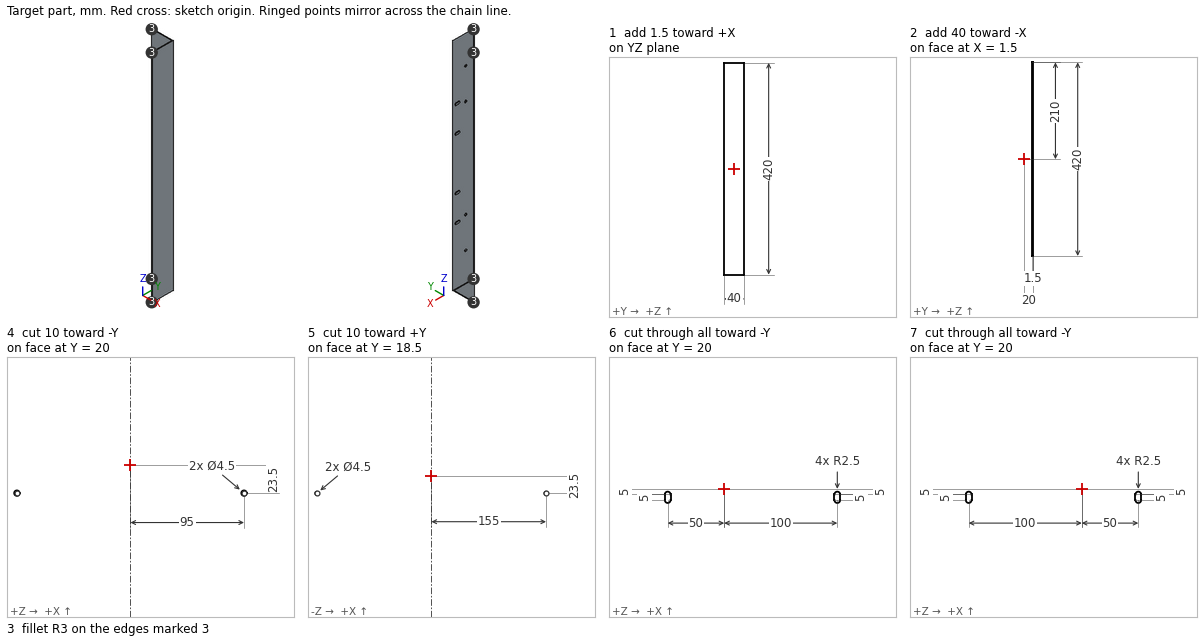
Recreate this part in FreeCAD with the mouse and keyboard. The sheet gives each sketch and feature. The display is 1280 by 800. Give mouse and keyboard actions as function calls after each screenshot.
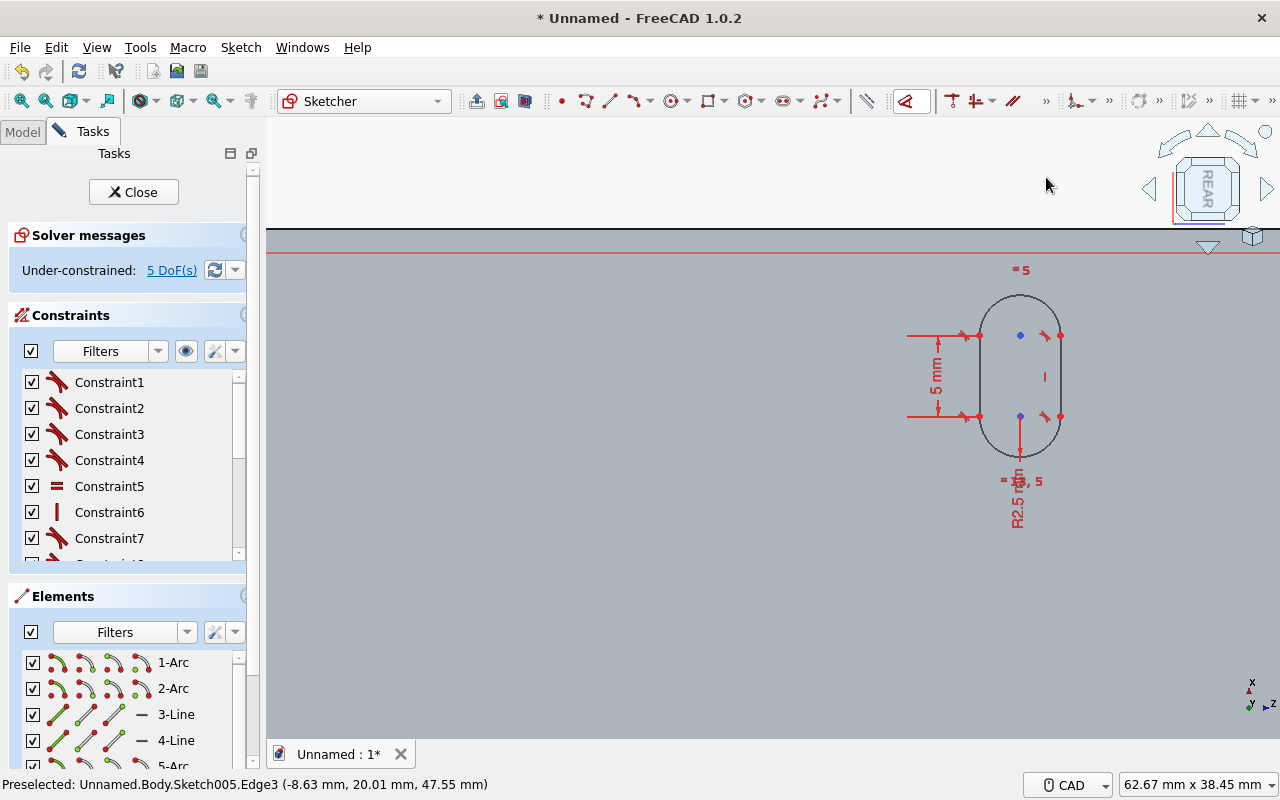
scroll(999, 452, down, 7)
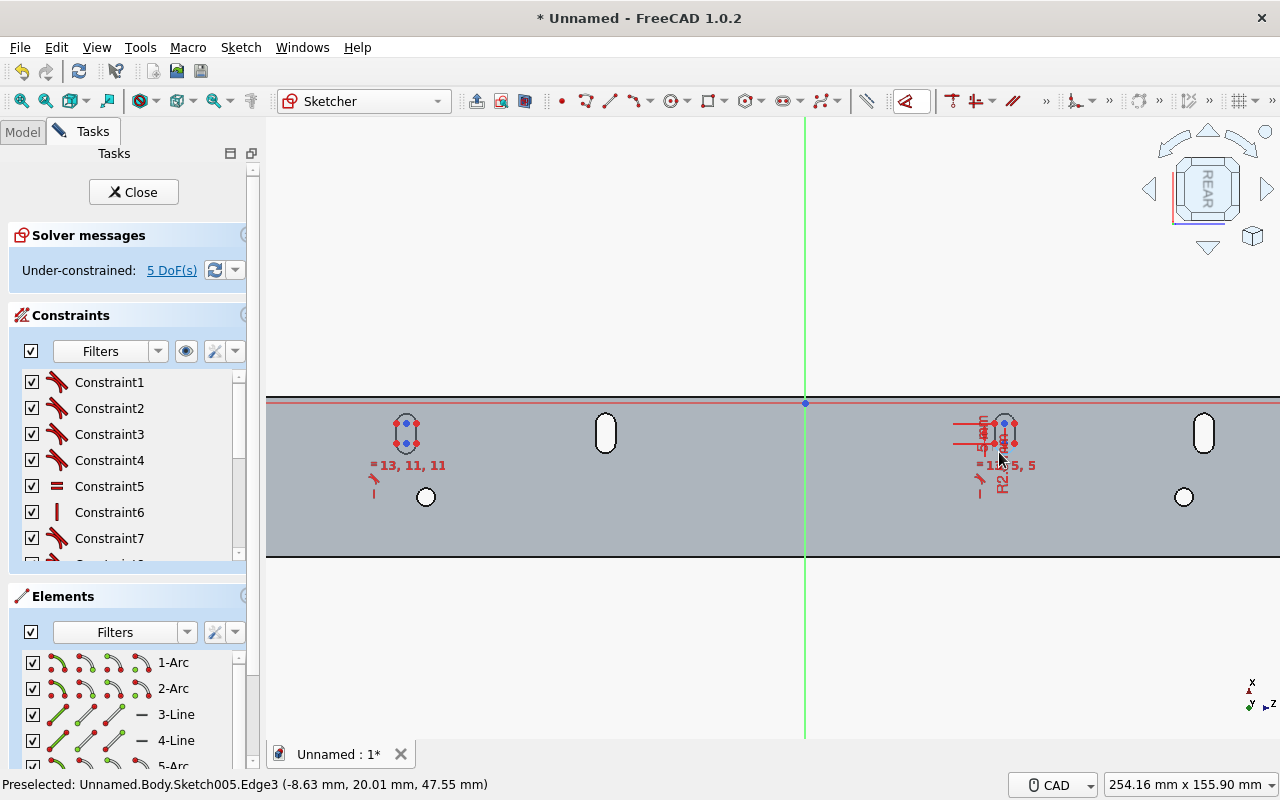
scroll(396, 438, up, 5)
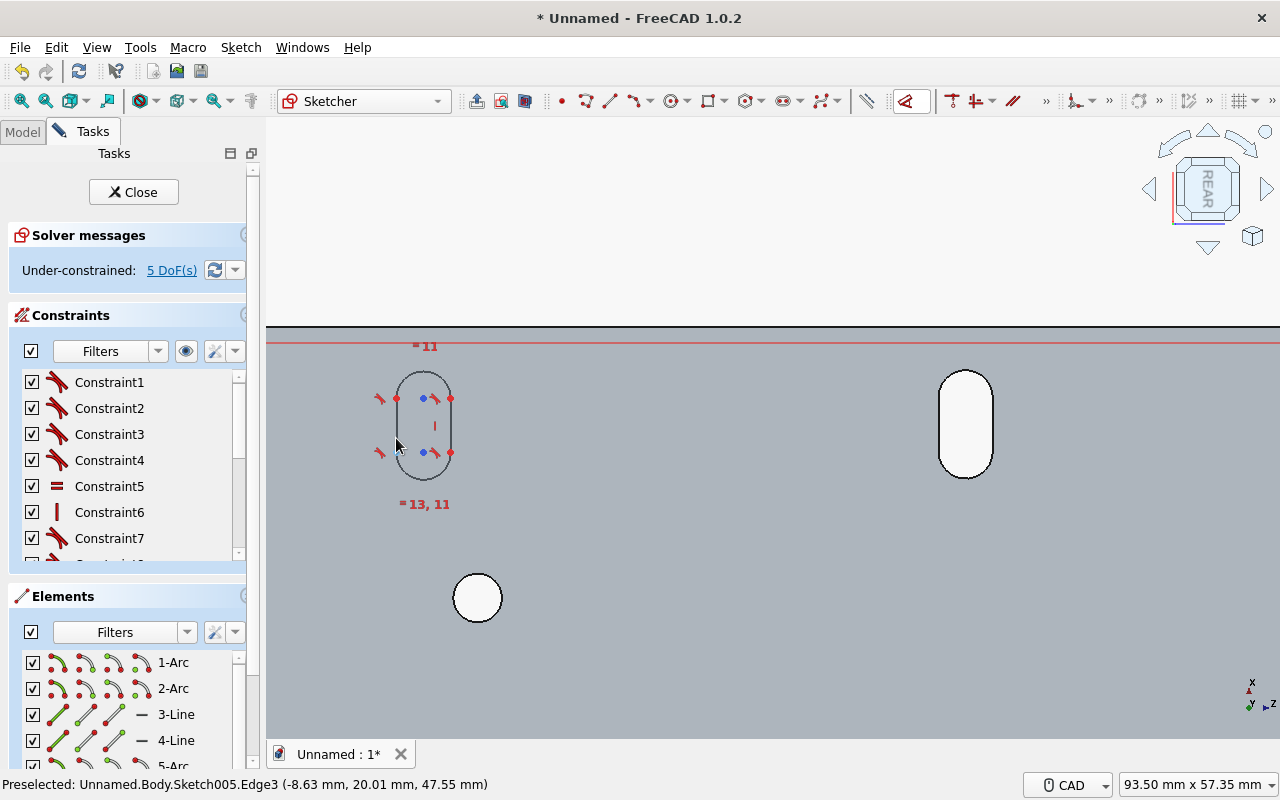
click(397, 436)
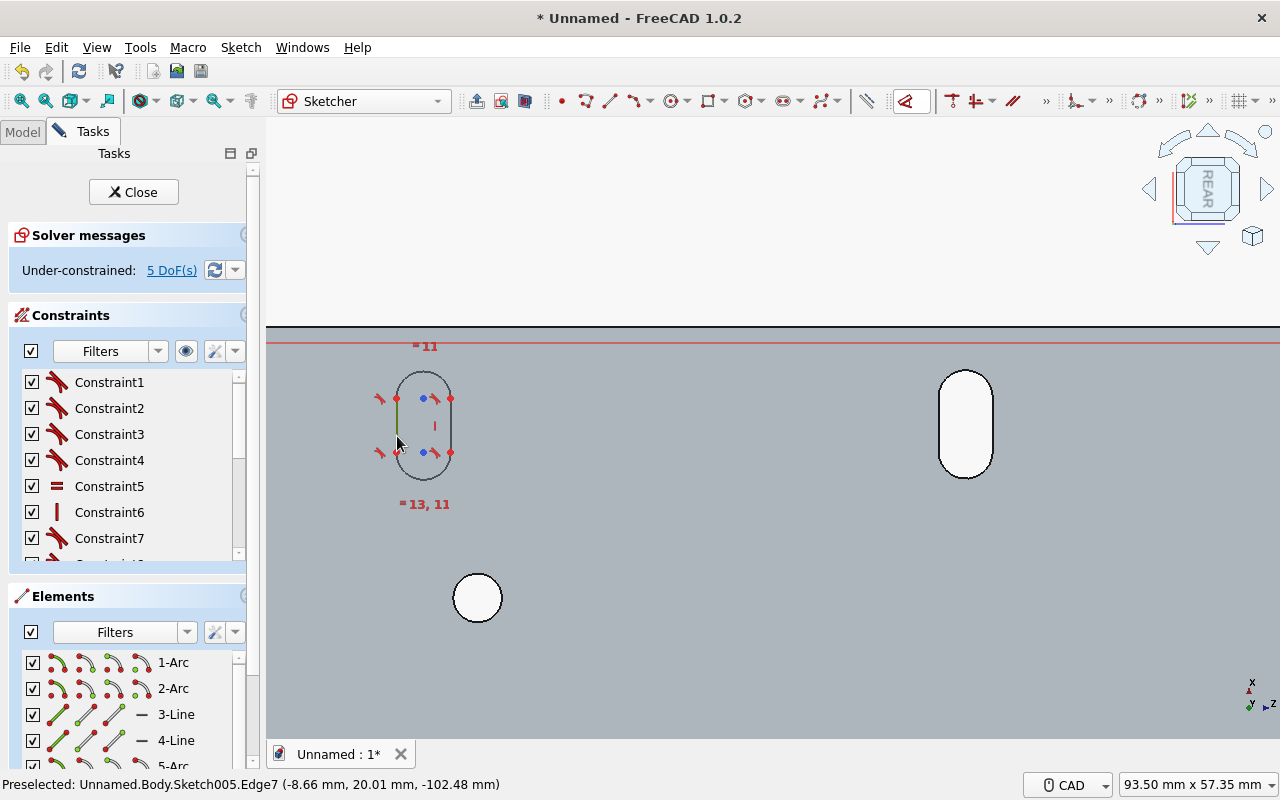
click(924, 102)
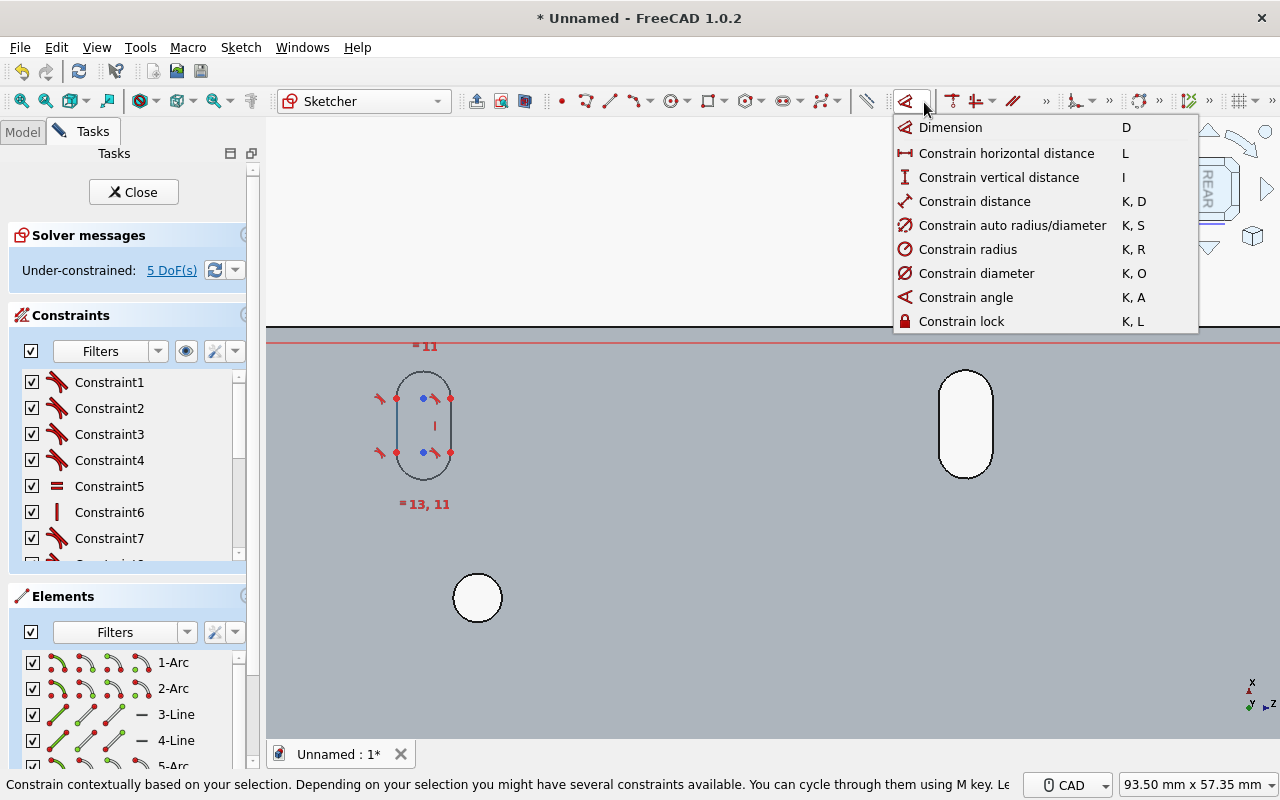
click(1046, 177)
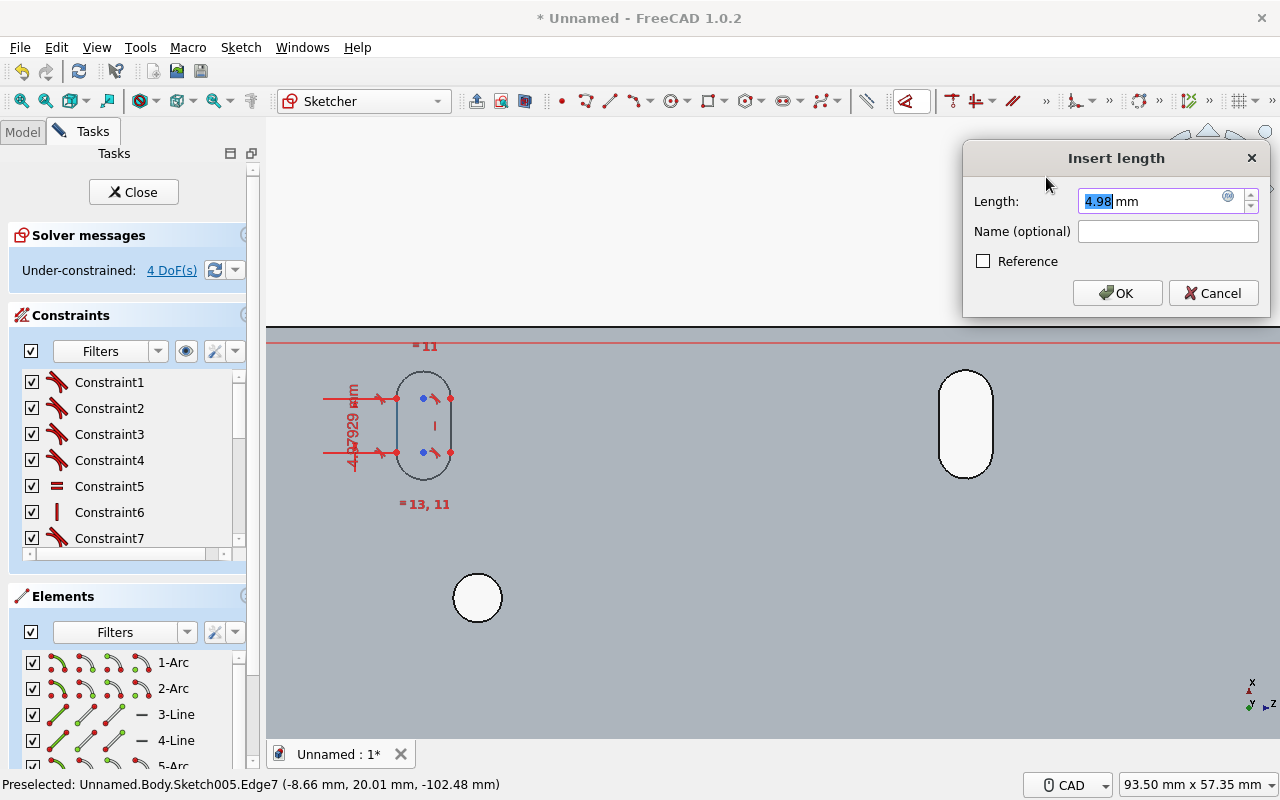
text(5)
key(Return)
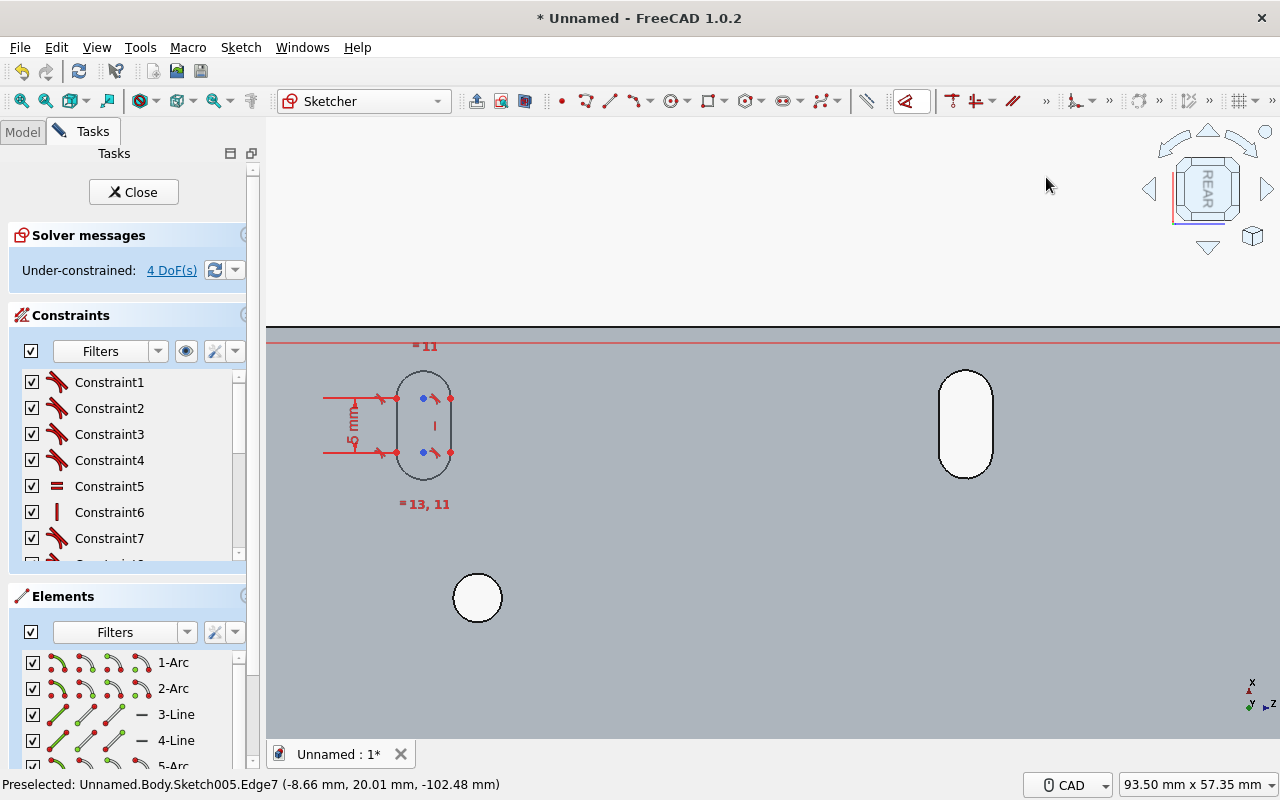
scroll(395, 438, down, 5)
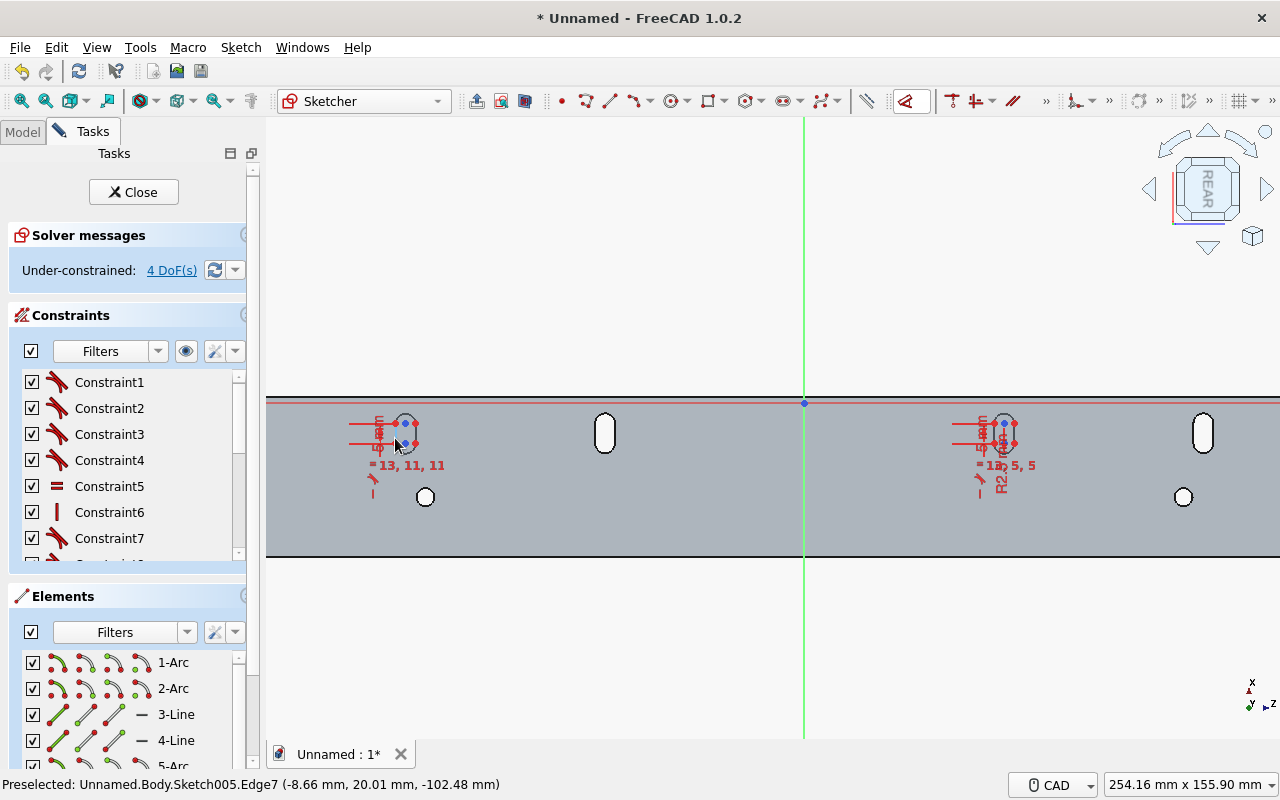
scroll(1014, 424, up, 4)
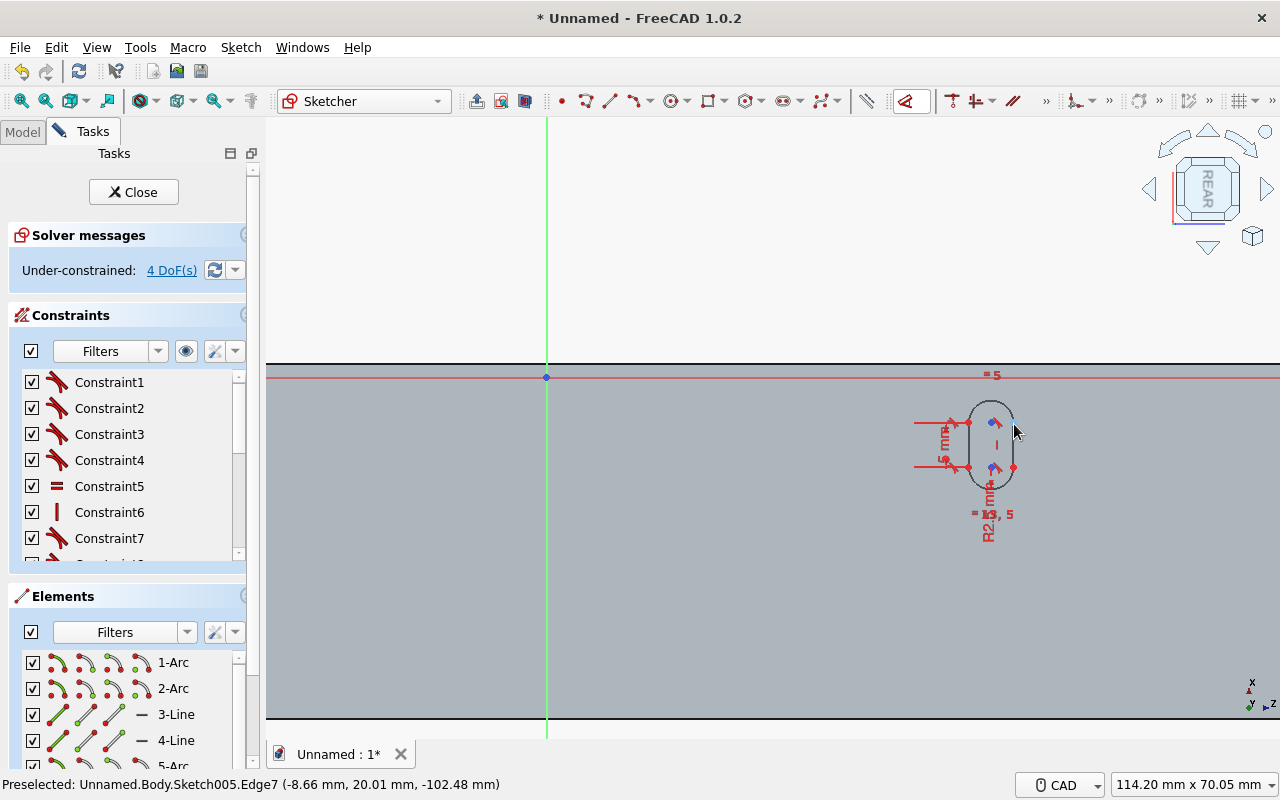
click(1013, 423)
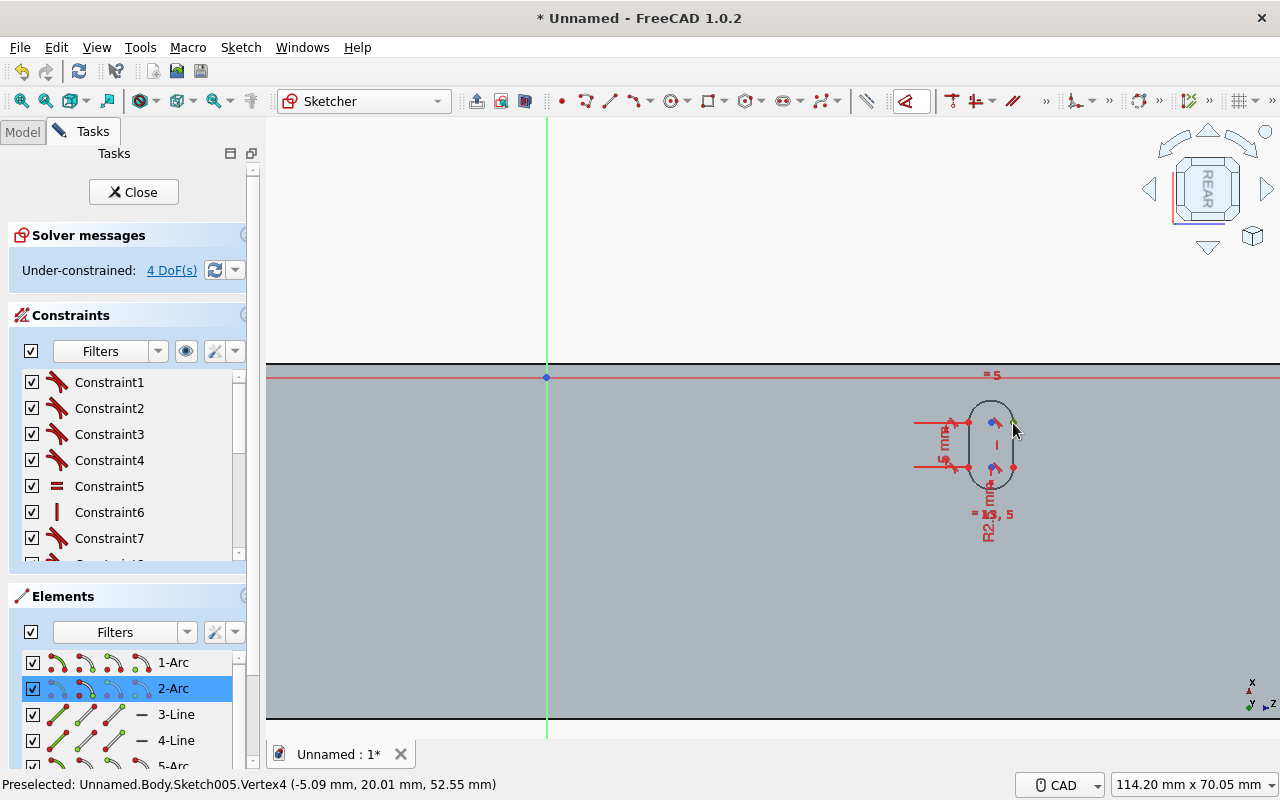
click(924, 102)